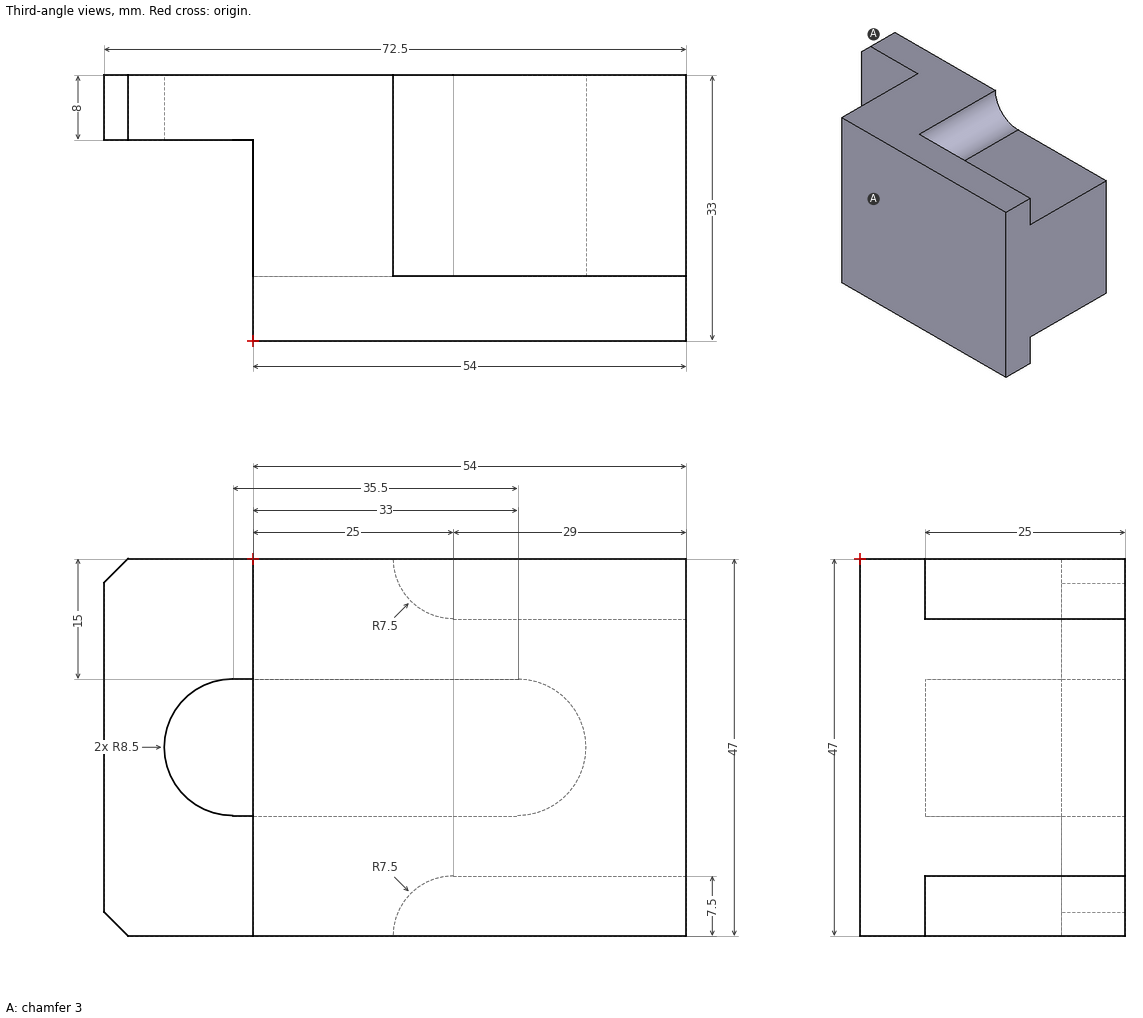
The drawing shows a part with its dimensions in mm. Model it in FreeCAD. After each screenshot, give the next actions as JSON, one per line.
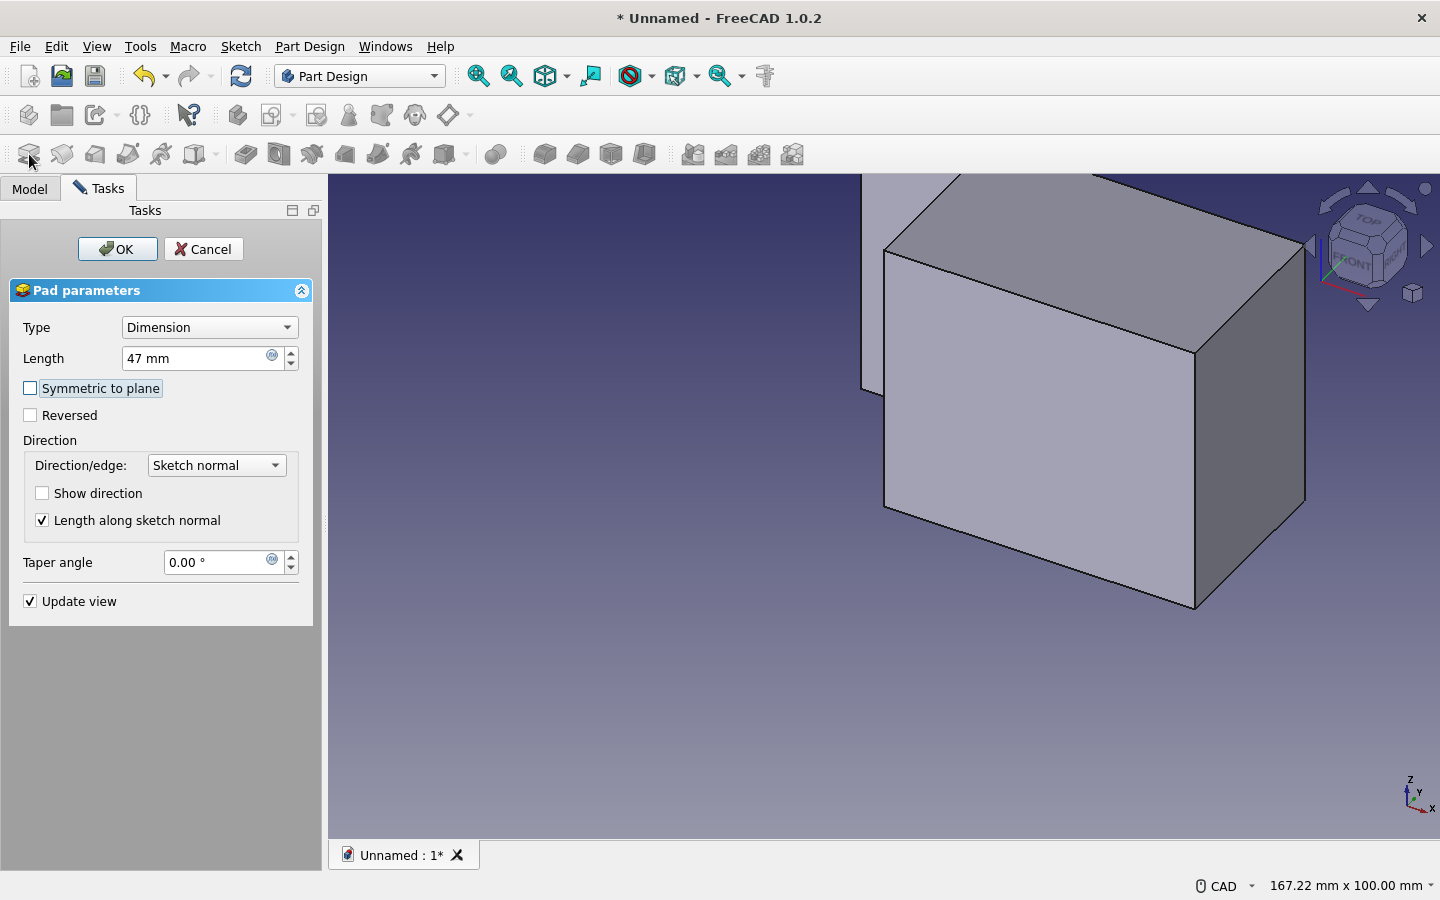
{"action": "left_click", "coordinate": [31, 415]}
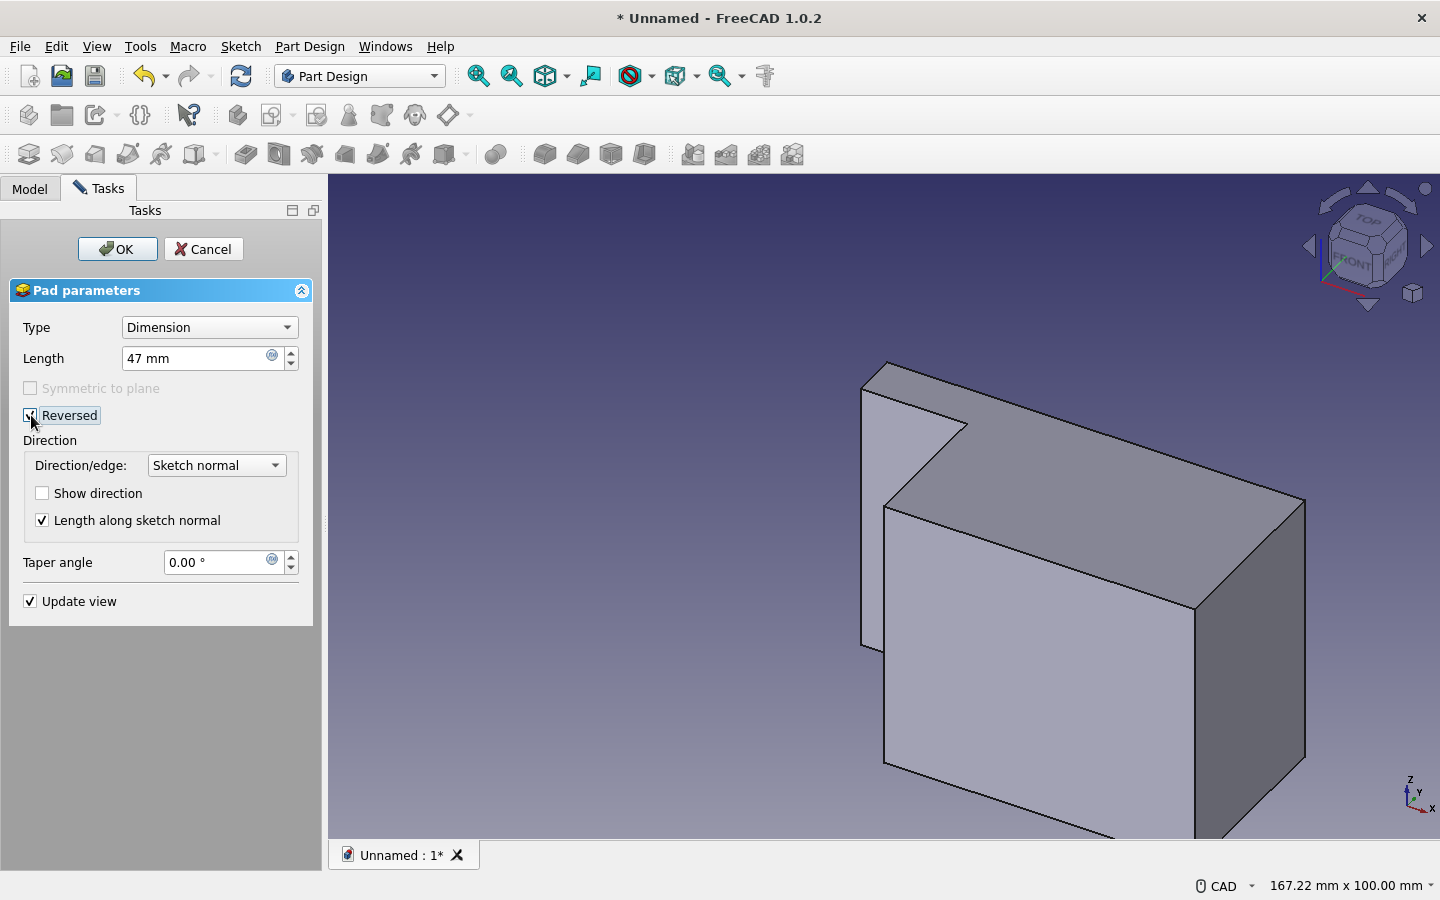
{"action": "left_click", "coordinate": [118, 249]}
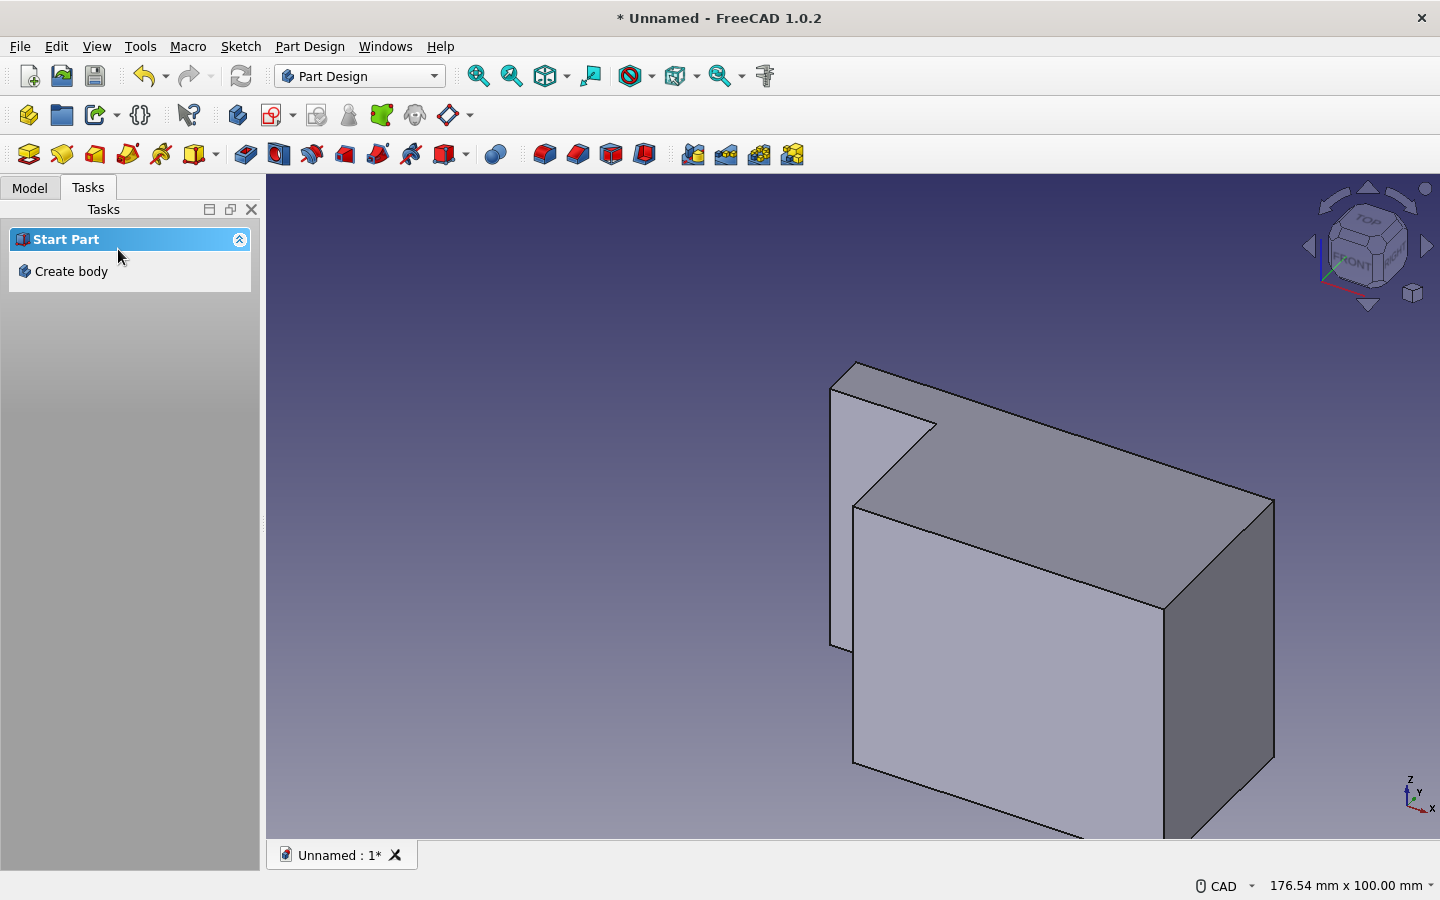
{"action": "left_click", "coordinate": [479, 76]}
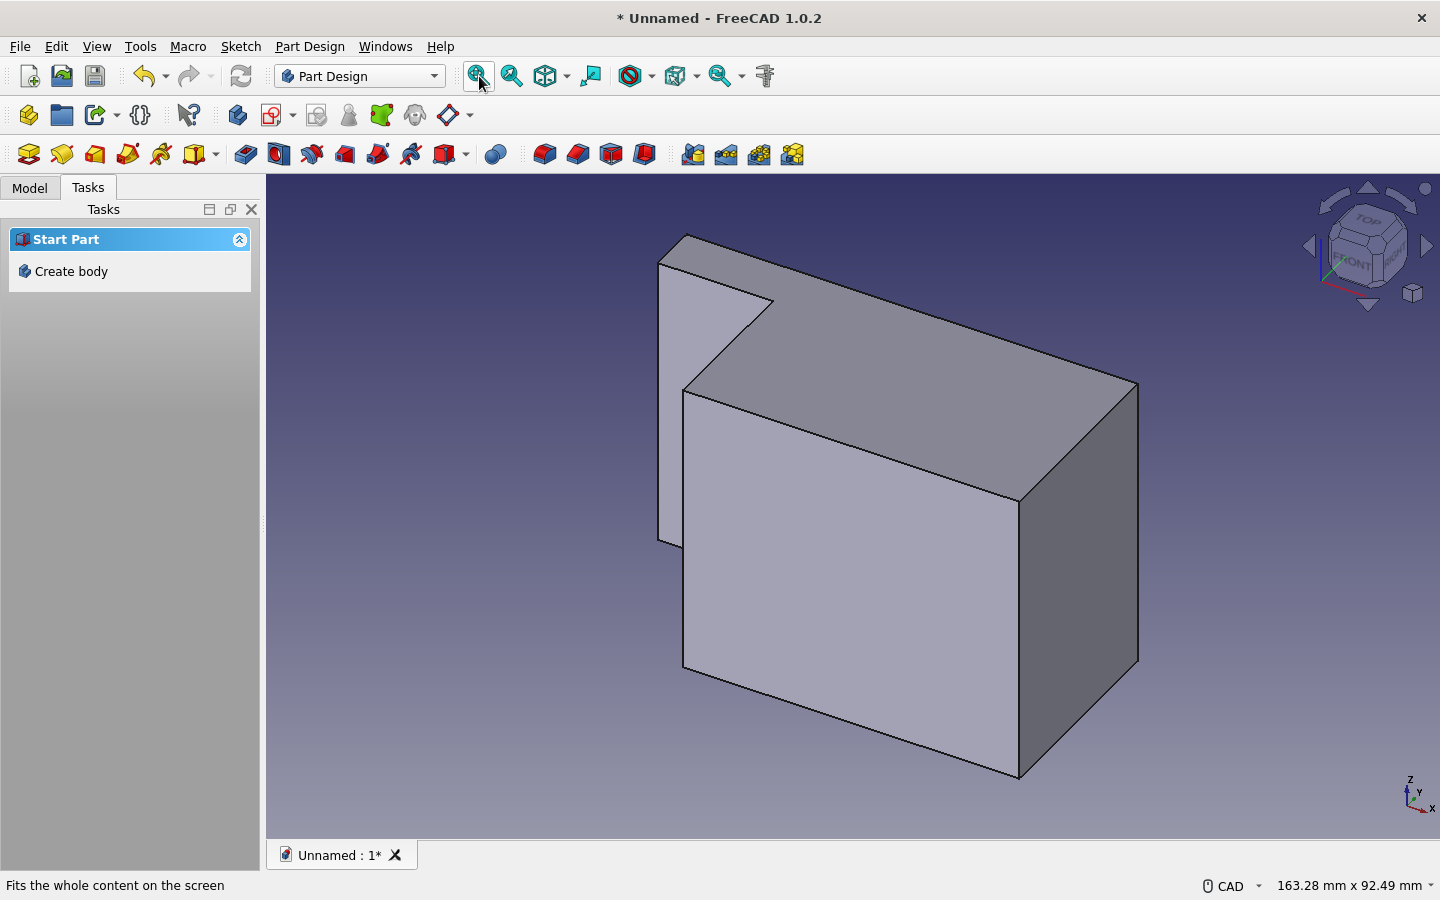
{"action": "key", "text": "4"}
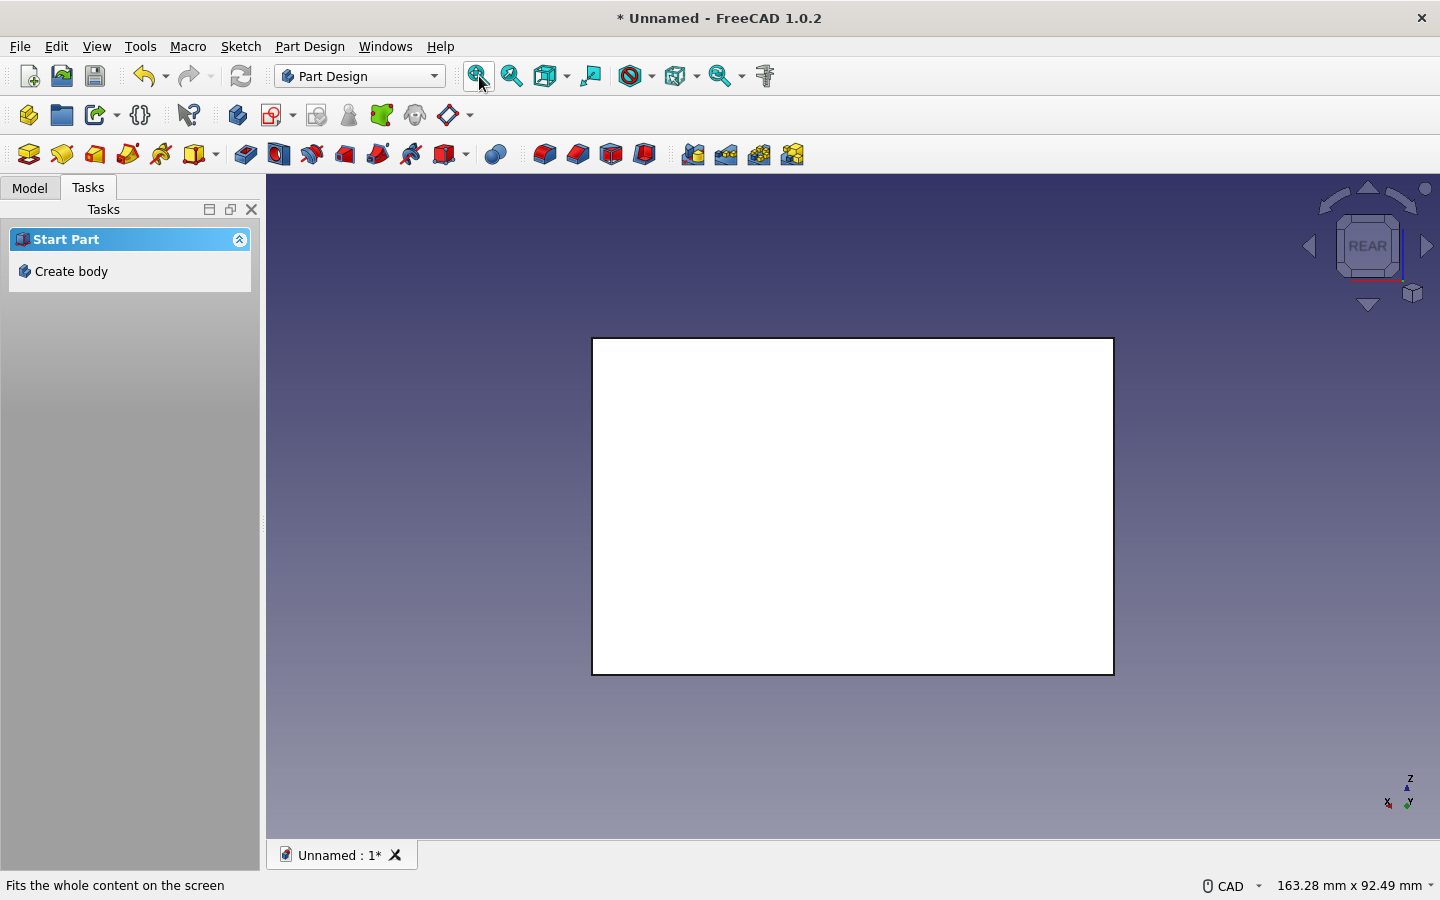
{"action": "left_click", "coordinate": [779, 505]}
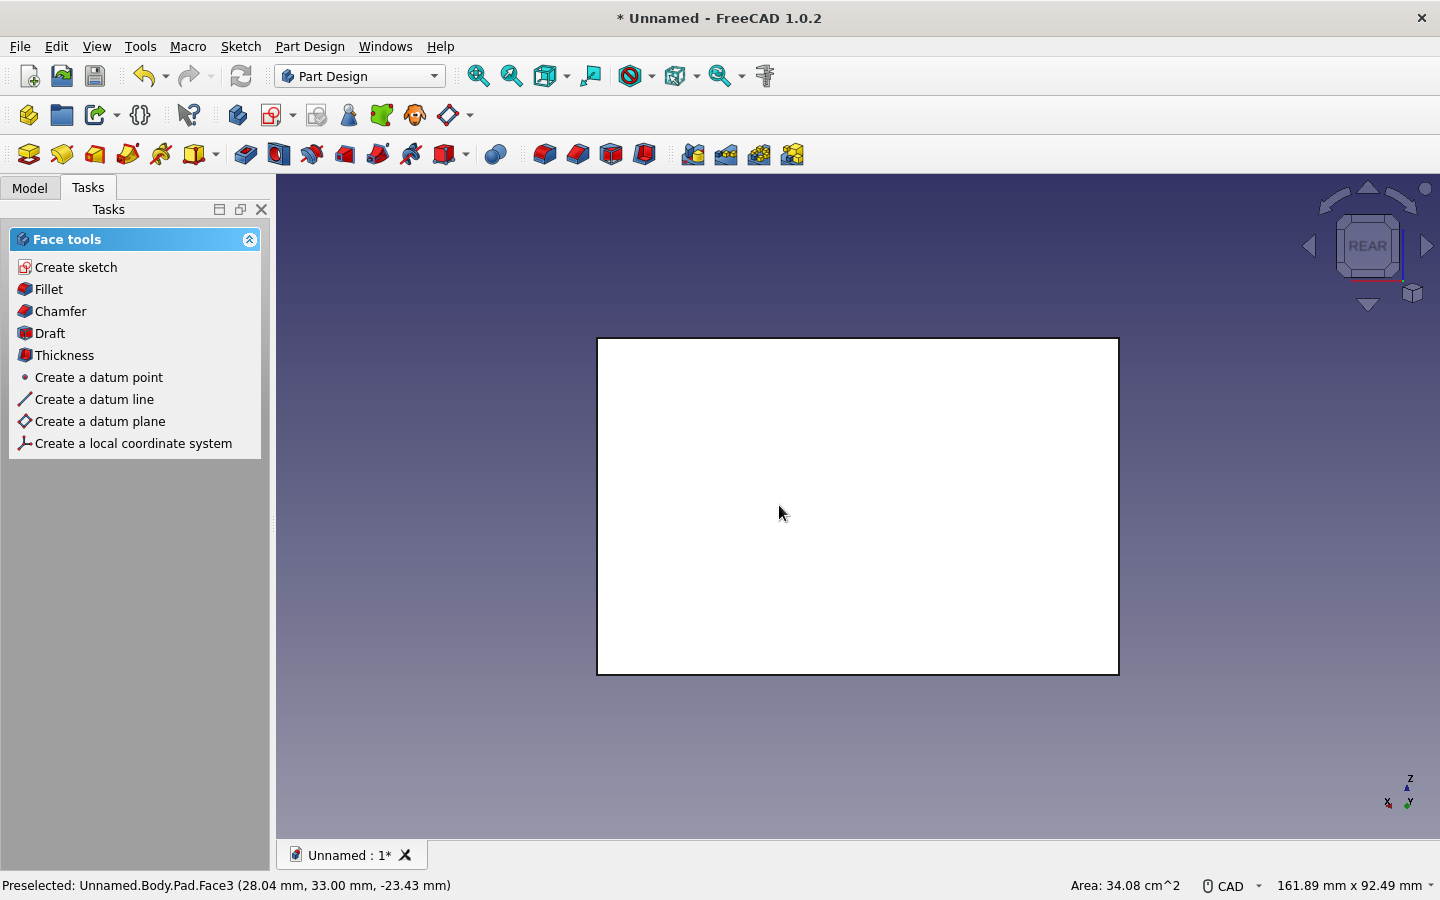
{"action": "left_click", "coordinate": [270, 116]}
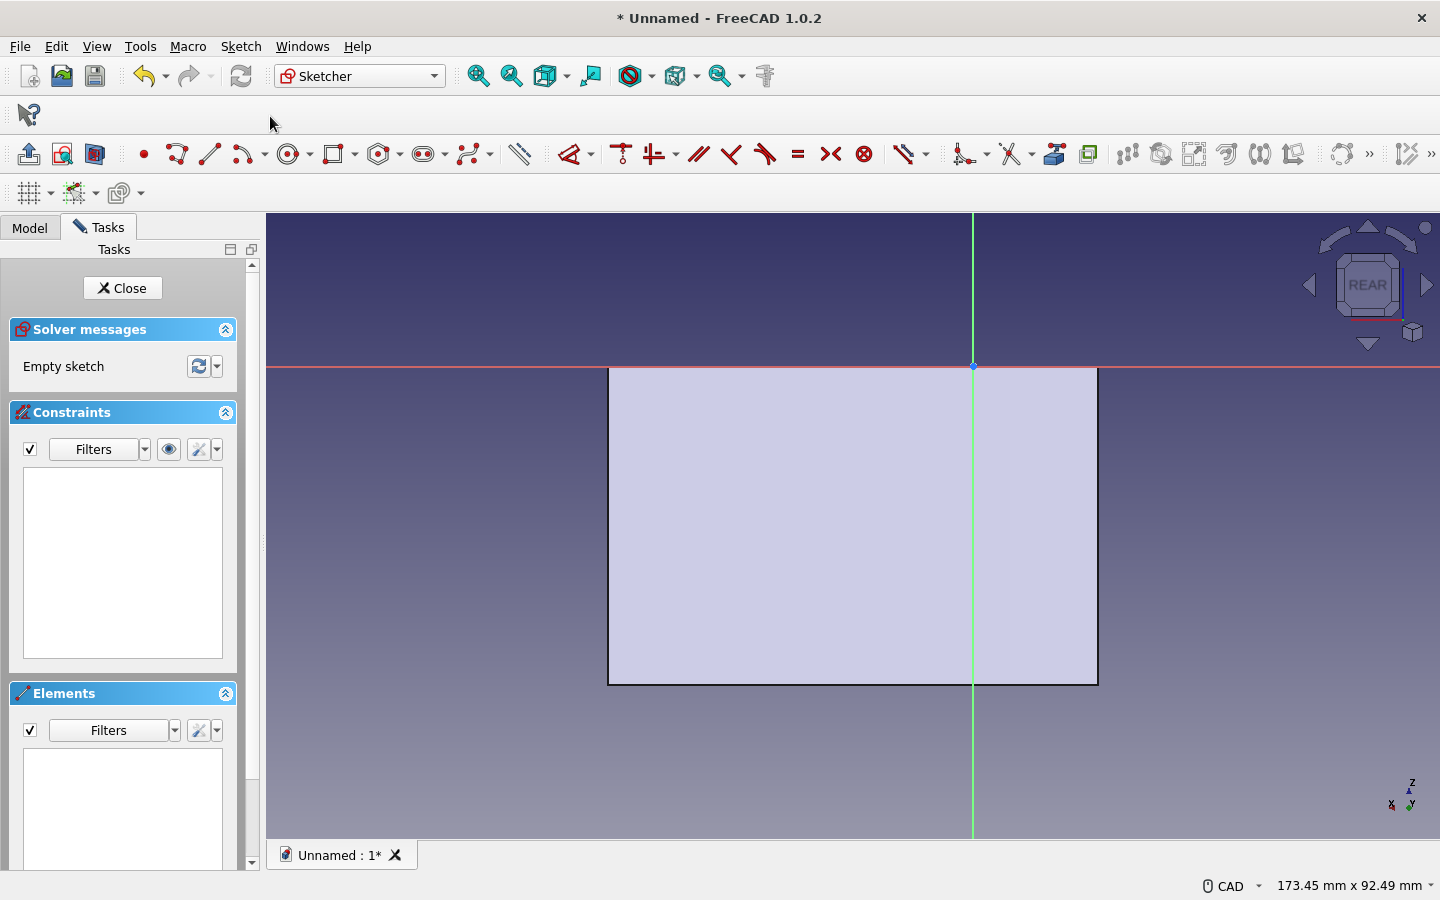
{"action": "scroll", "coordinate": [798, 241], "scroll_direction": "up", "scroll_amount": 3}